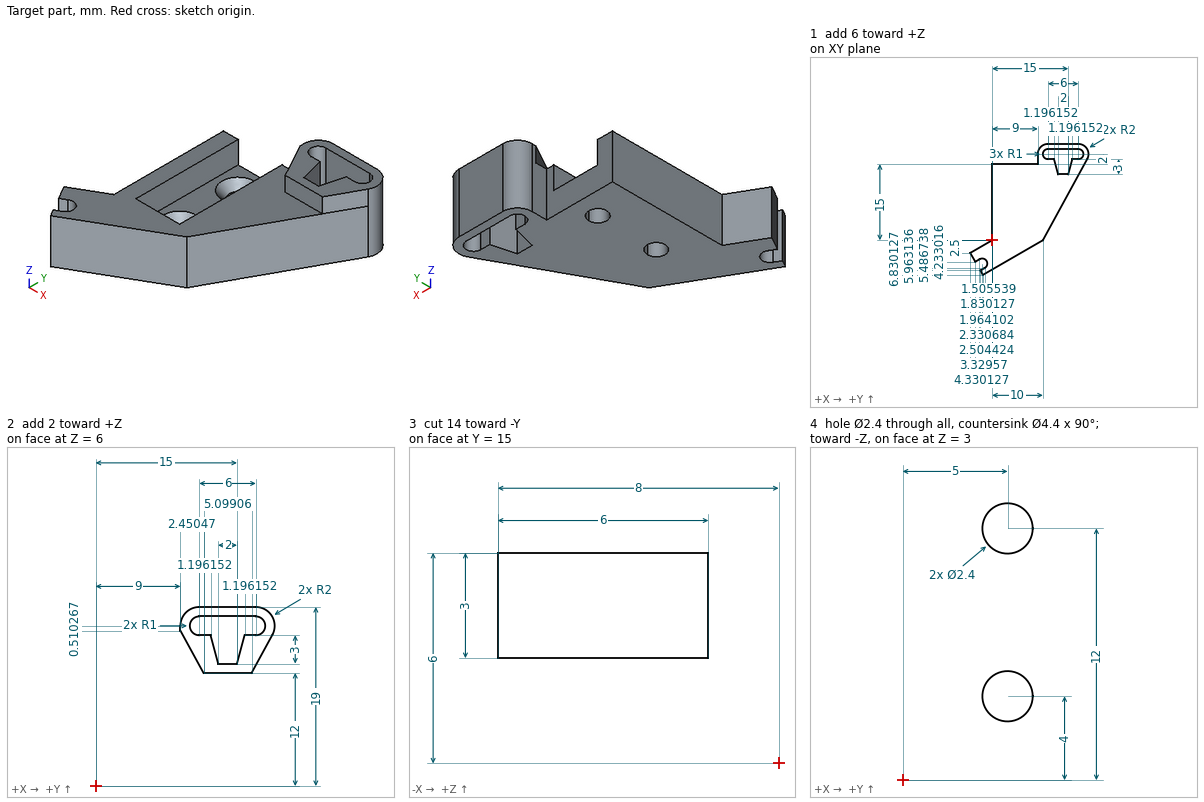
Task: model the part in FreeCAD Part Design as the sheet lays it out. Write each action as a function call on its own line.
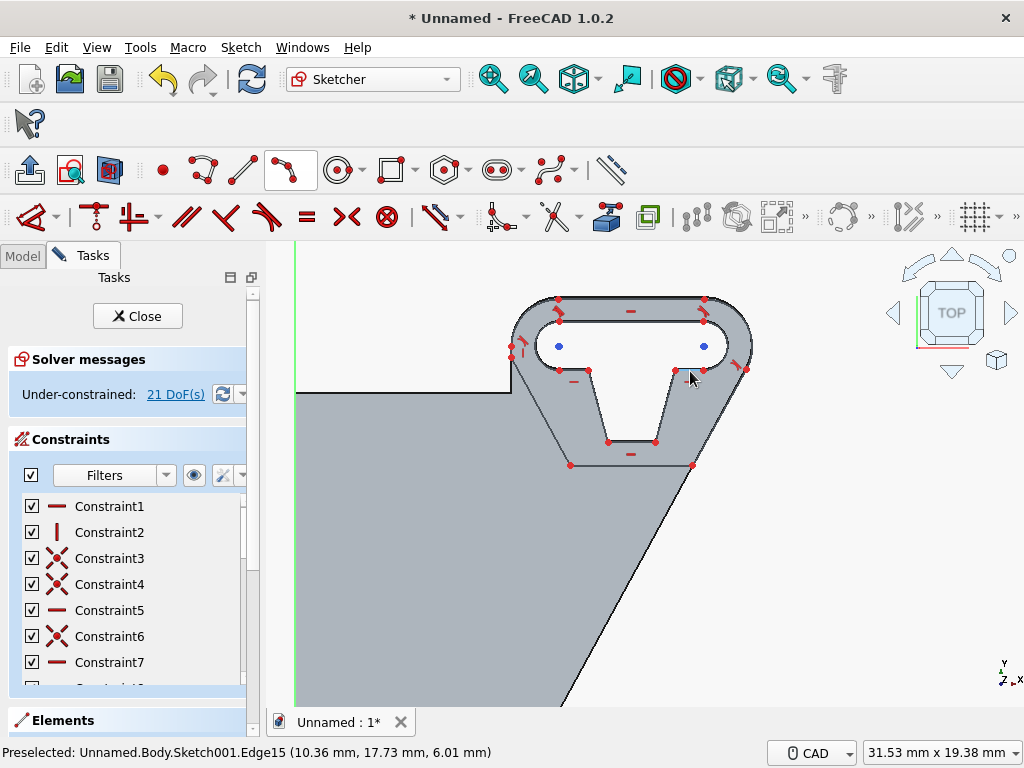
click(689, 370)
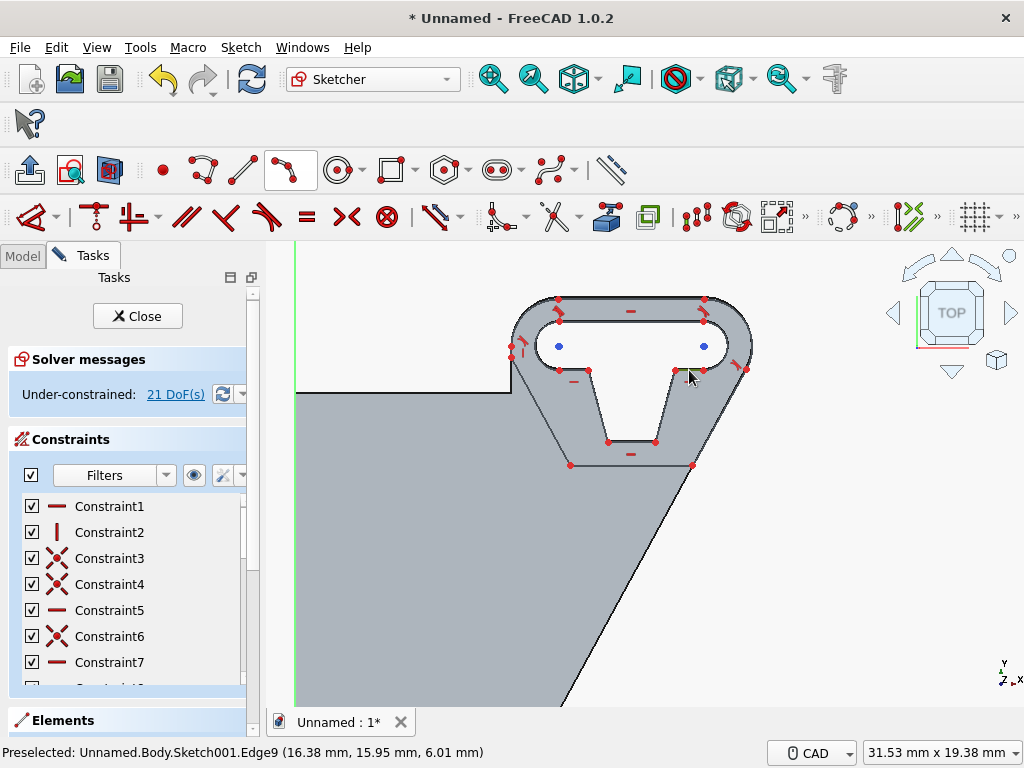
click(723, 360)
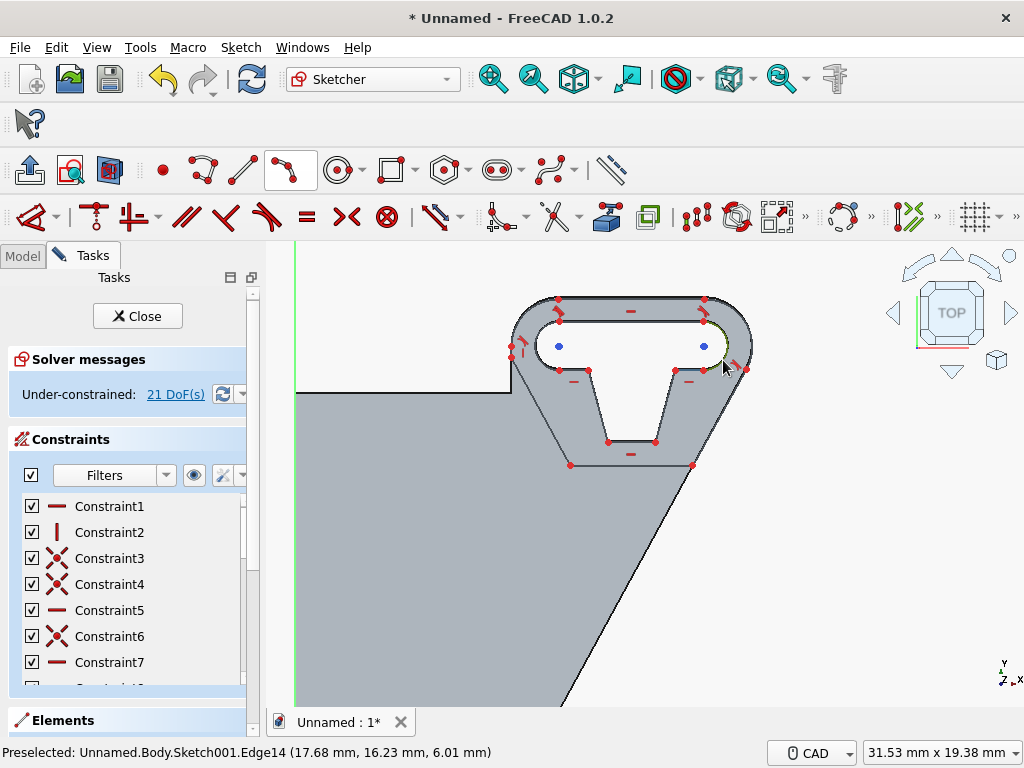
key(t)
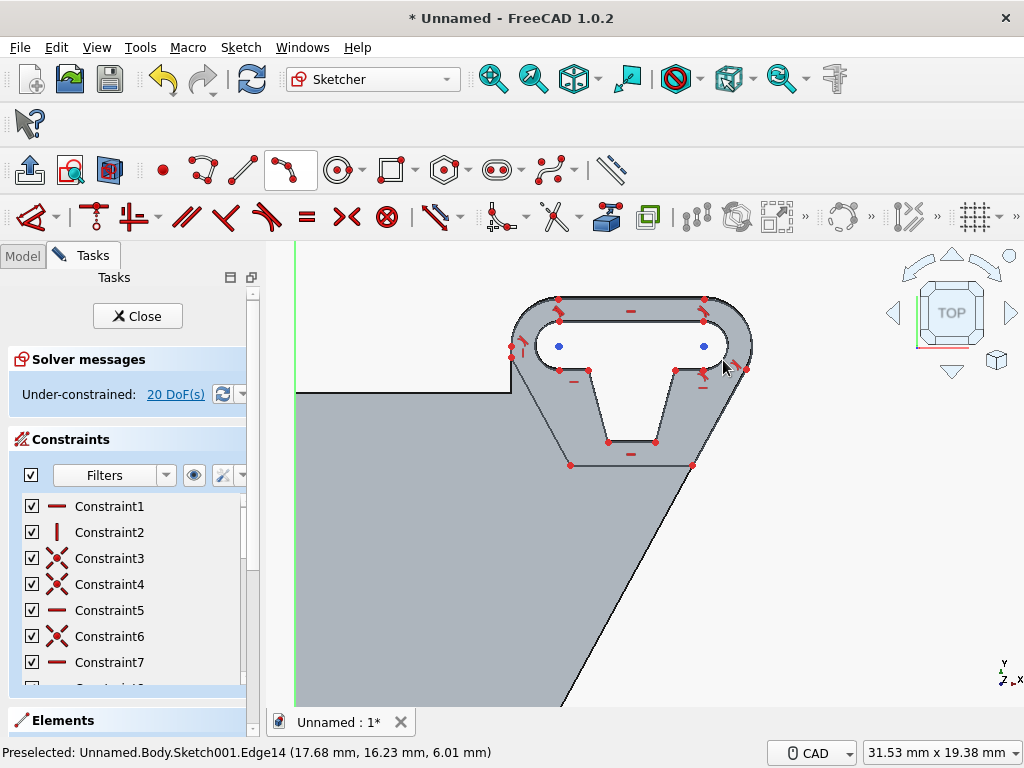
click(577, 370)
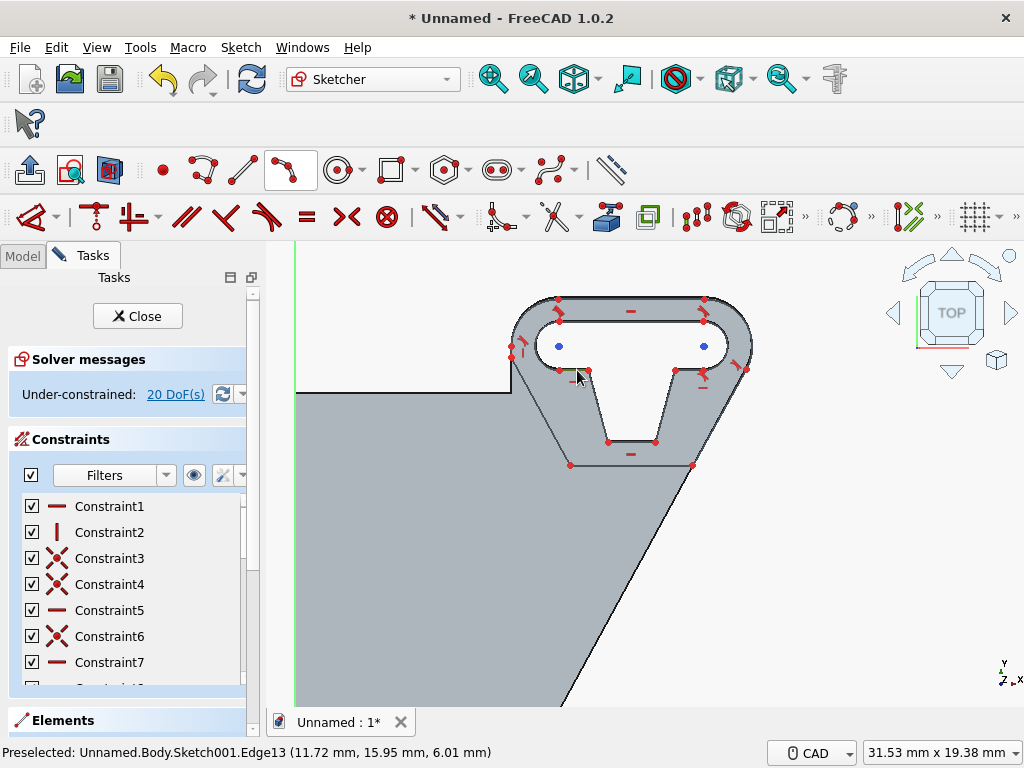
click(540, 332)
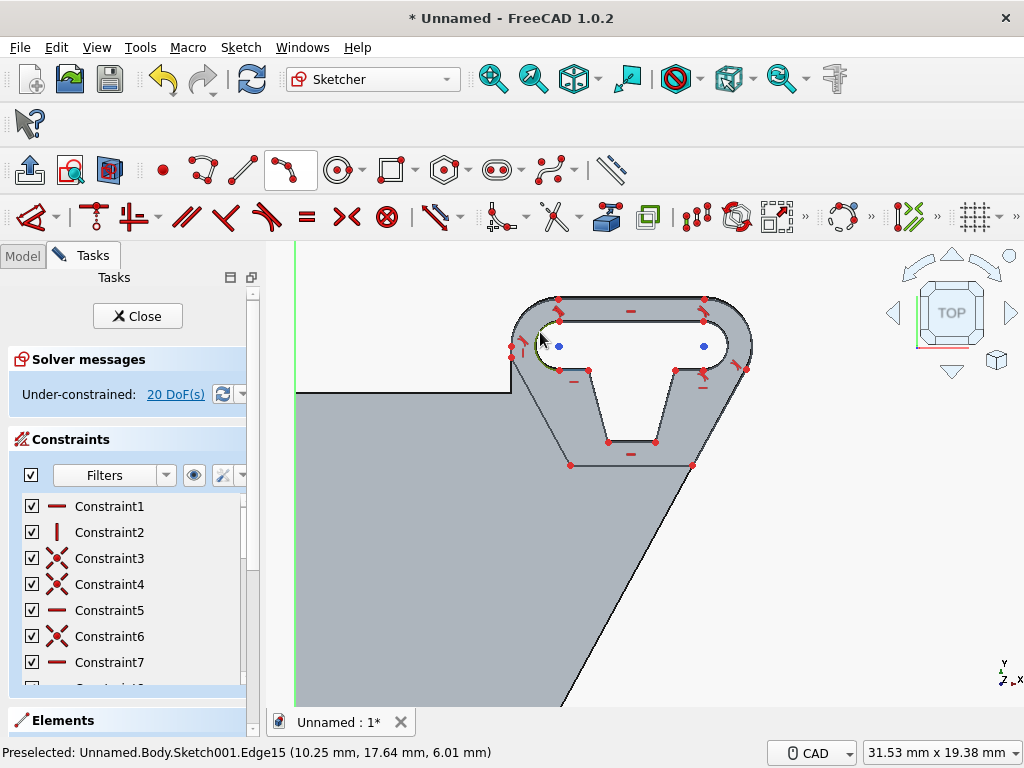
key(t)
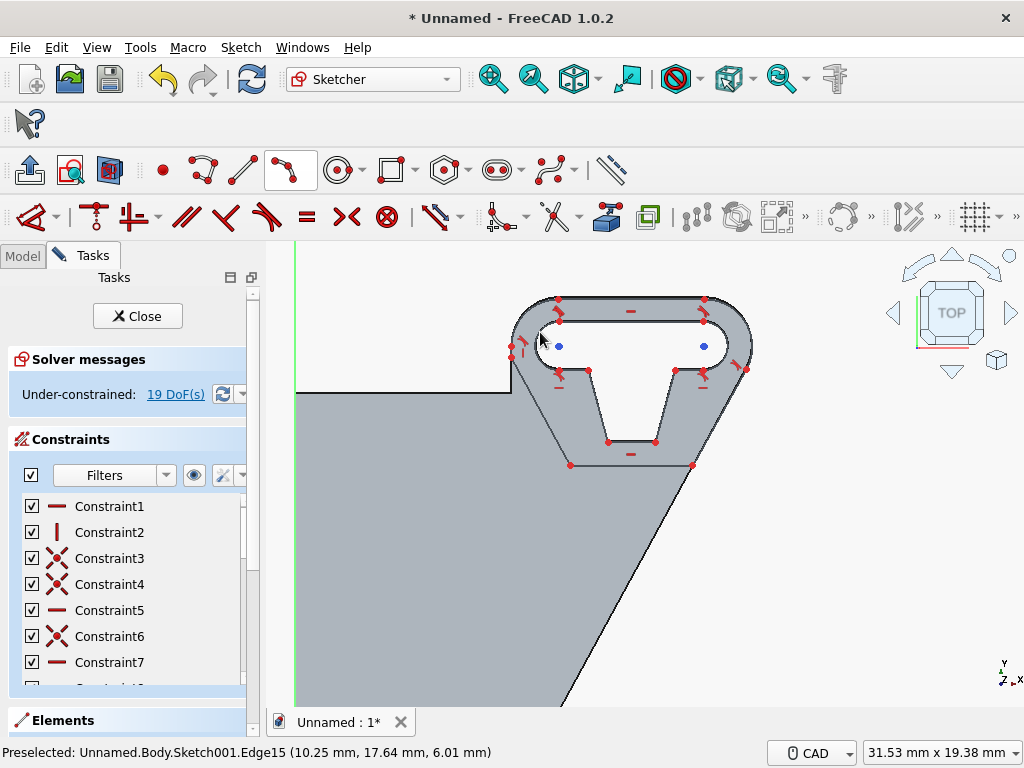
click(752, 341)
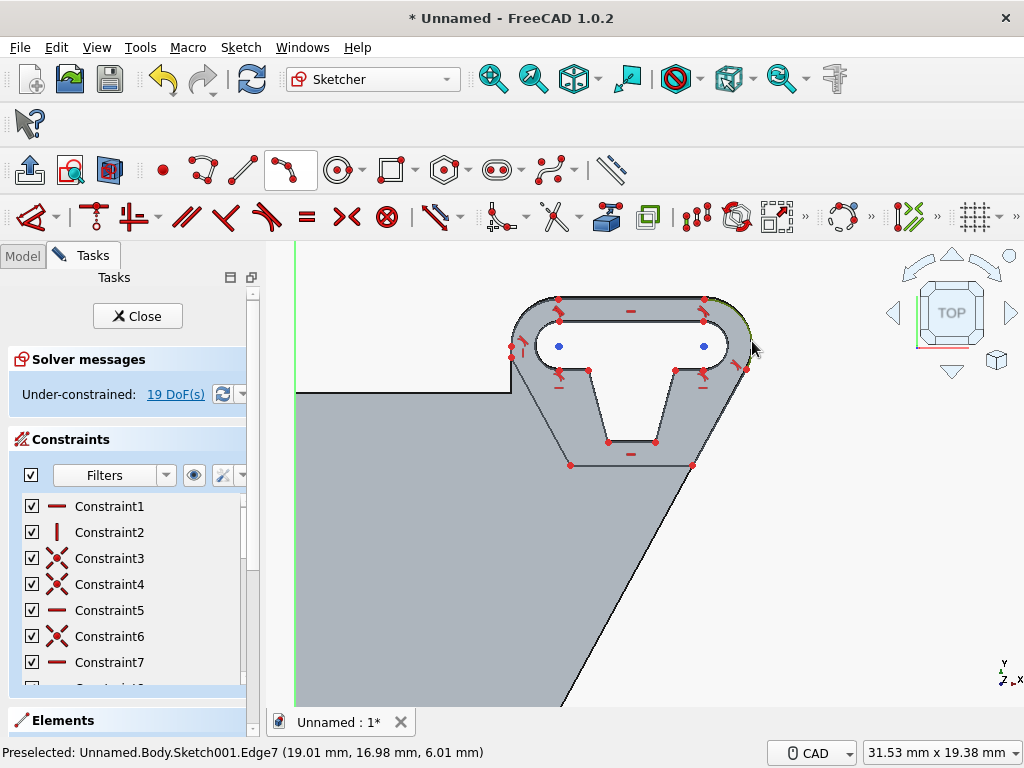
click(723, 360)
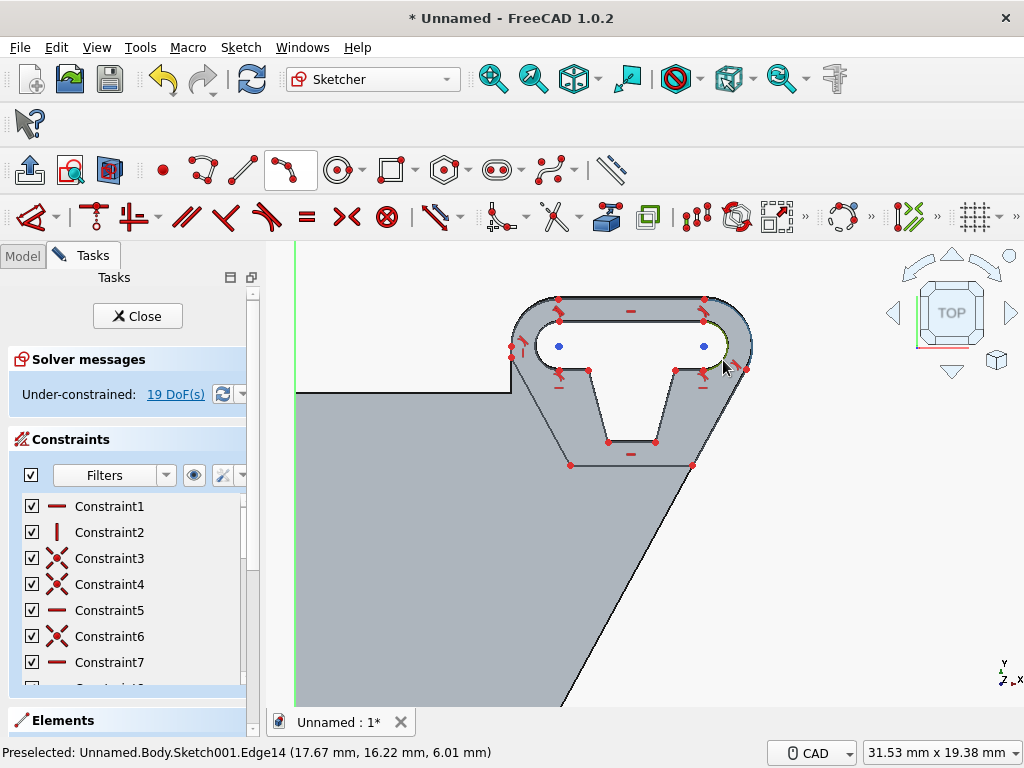
key(c)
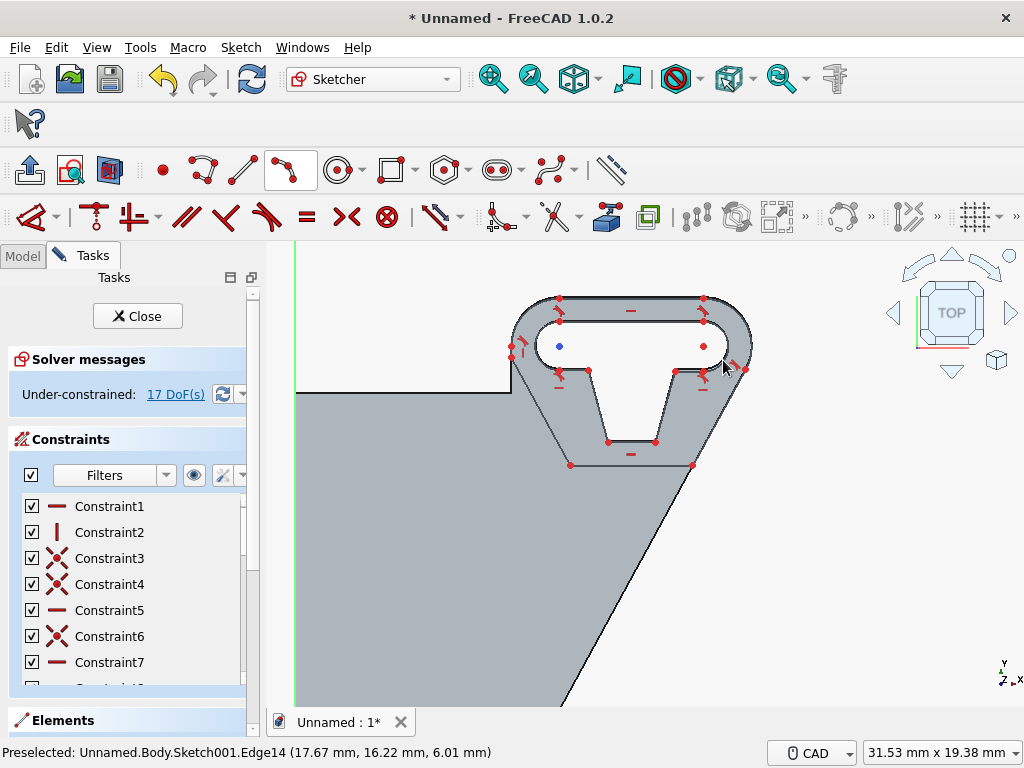
click(538, 304)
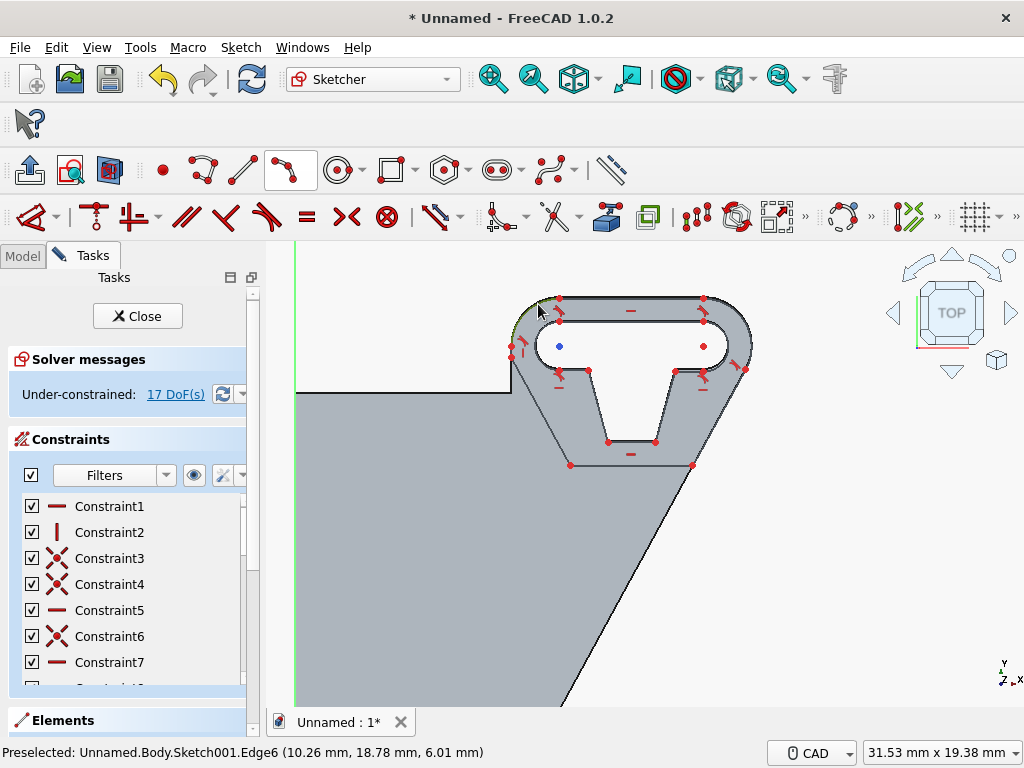
click(540, 332)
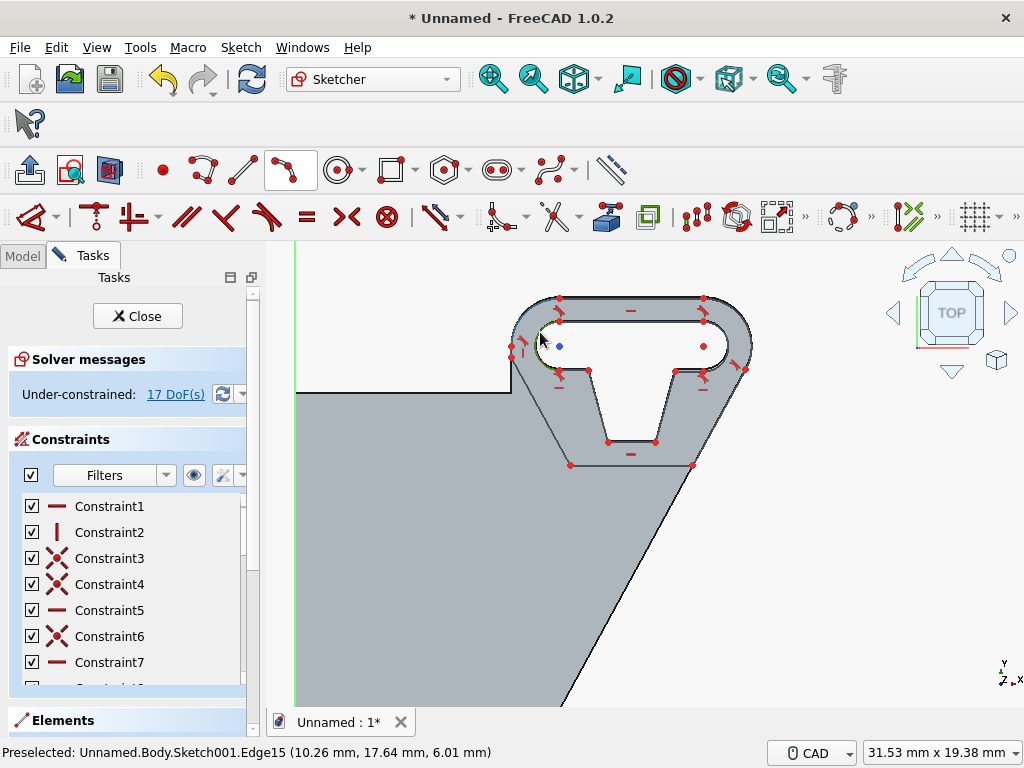
key(c)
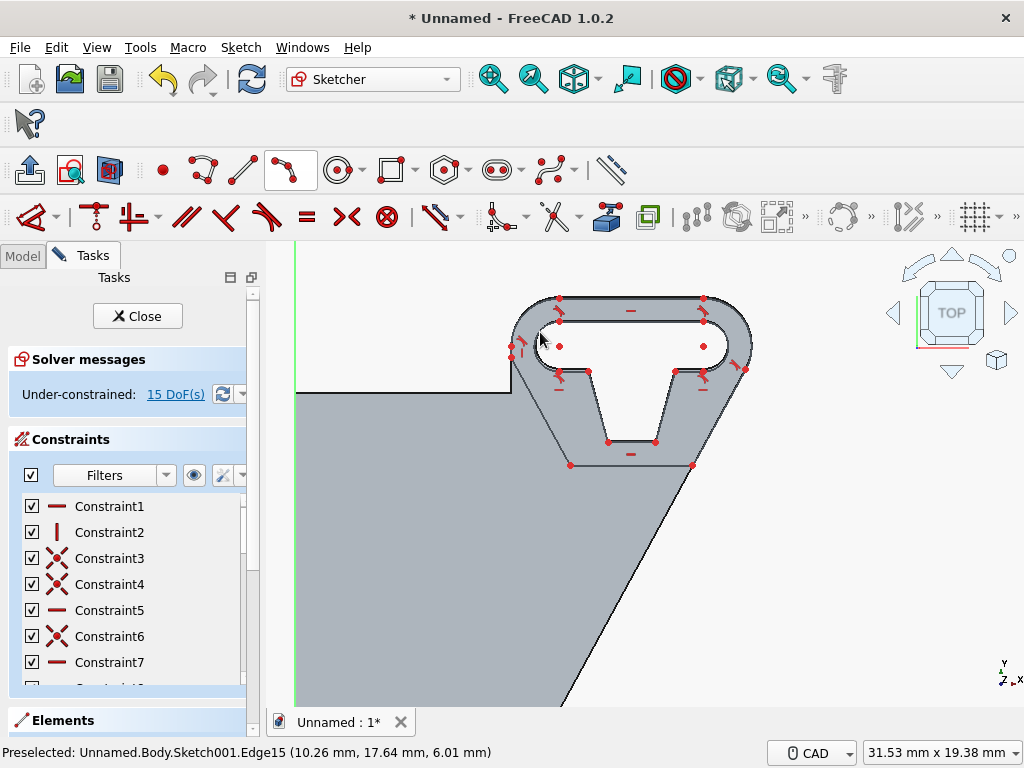
click(537, 304)